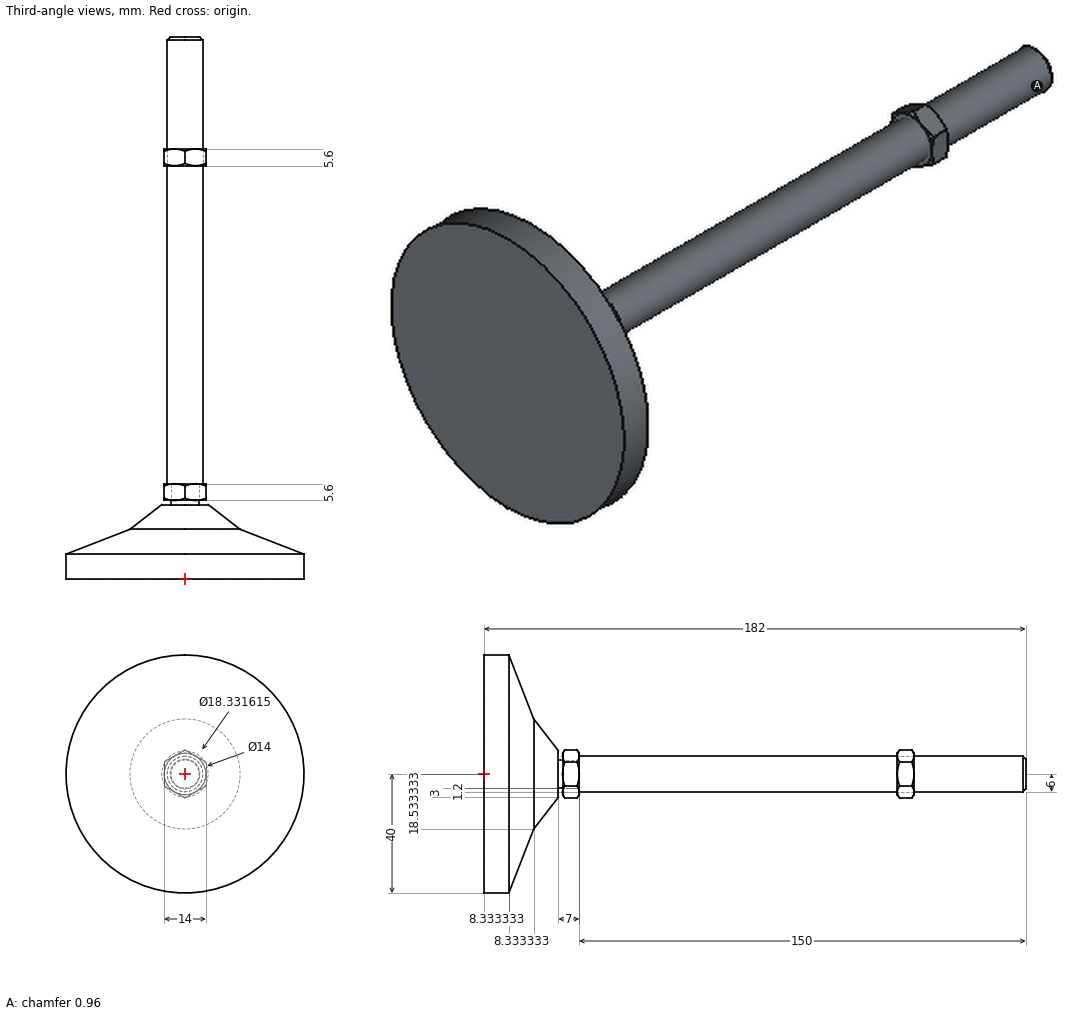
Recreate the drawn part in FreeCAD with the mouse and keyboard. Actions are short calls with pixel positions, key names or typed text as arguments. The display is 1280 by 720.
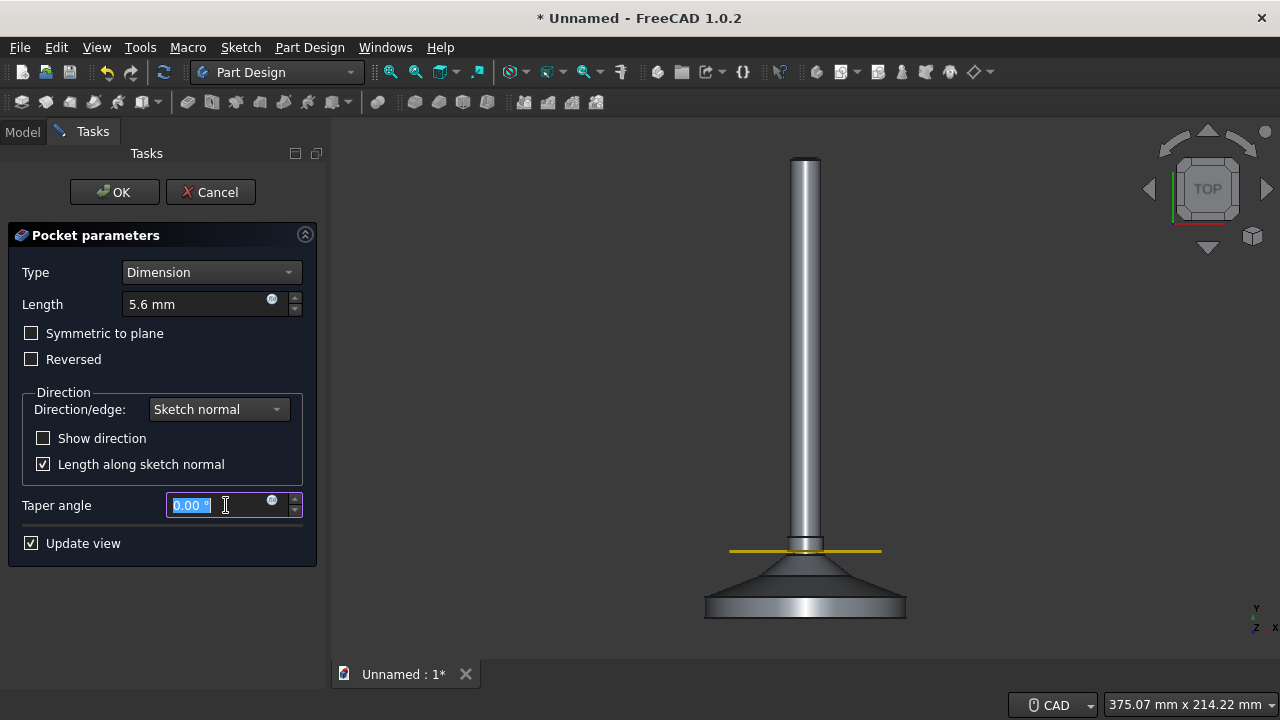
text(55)
key(Tab)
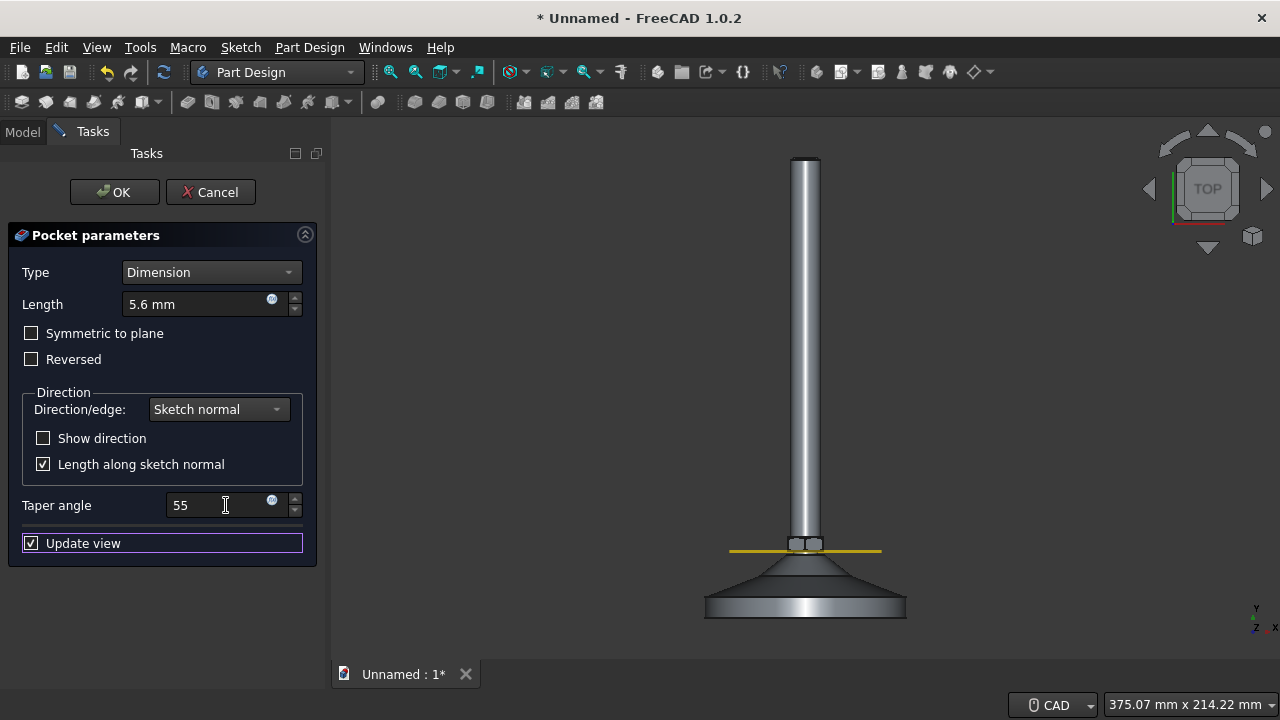
click(115, 192)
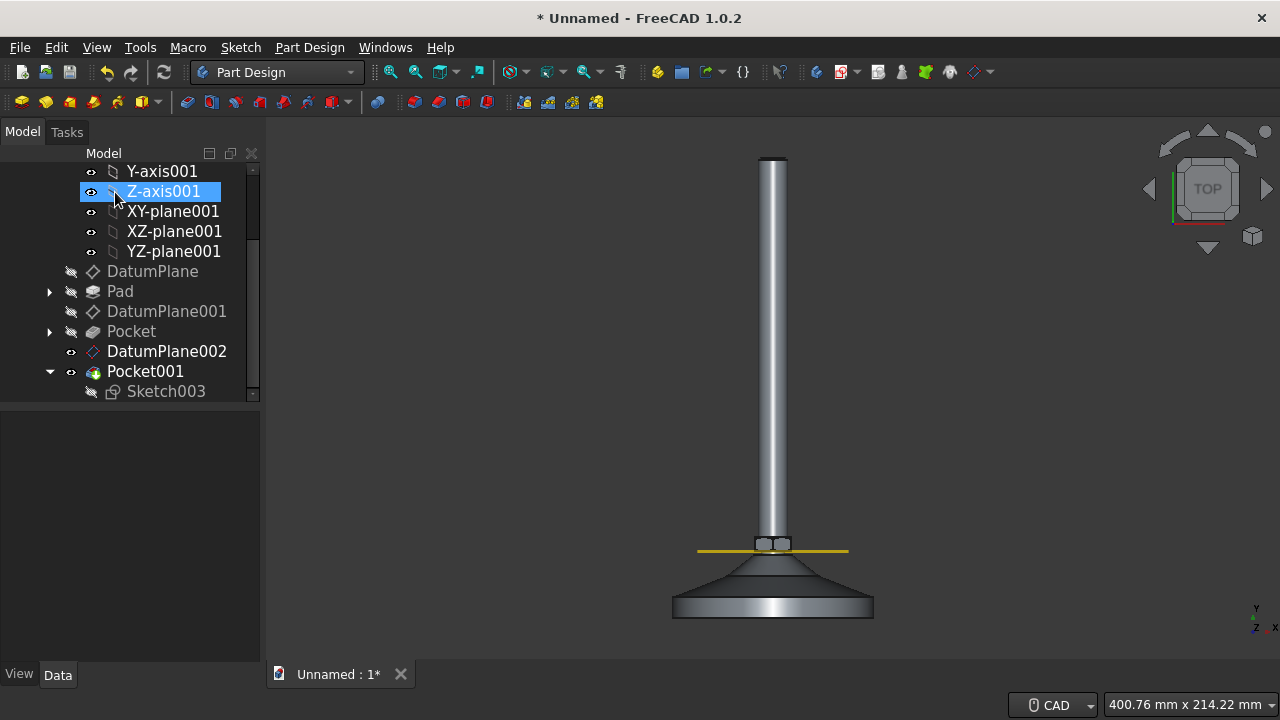
click(116, 352)
key(space)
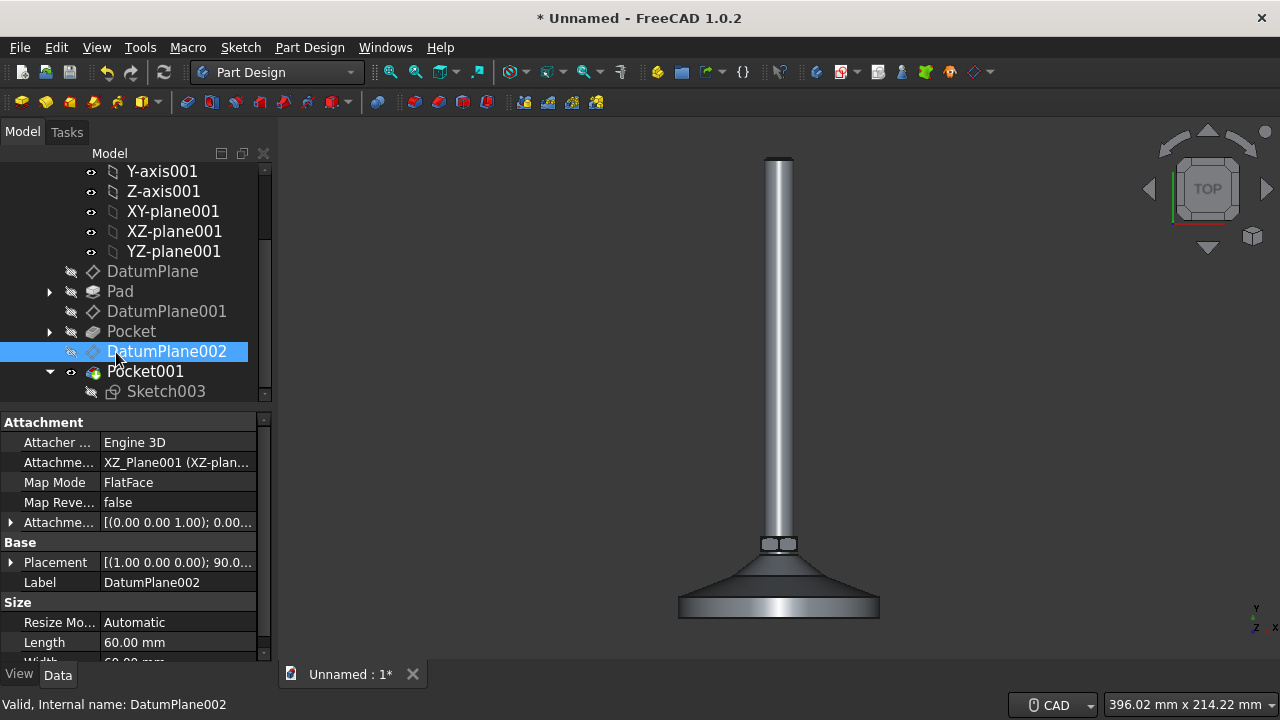
click(392, 72)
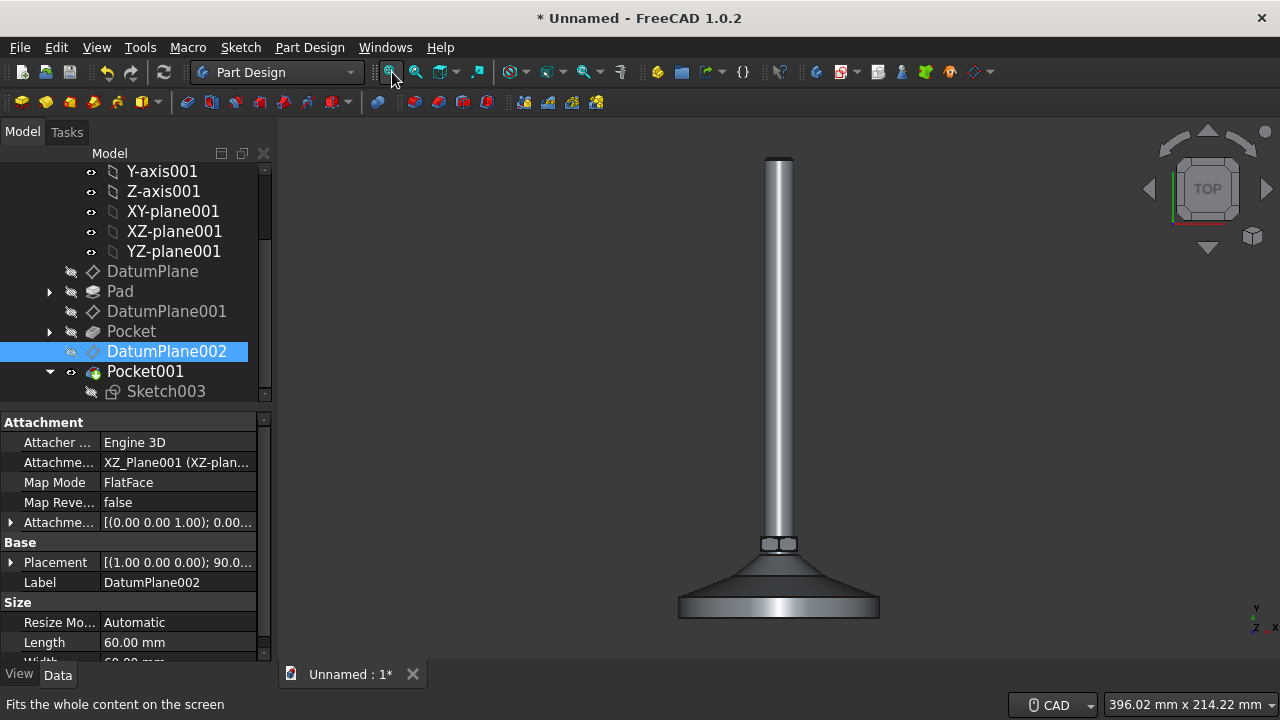
click(318, 619)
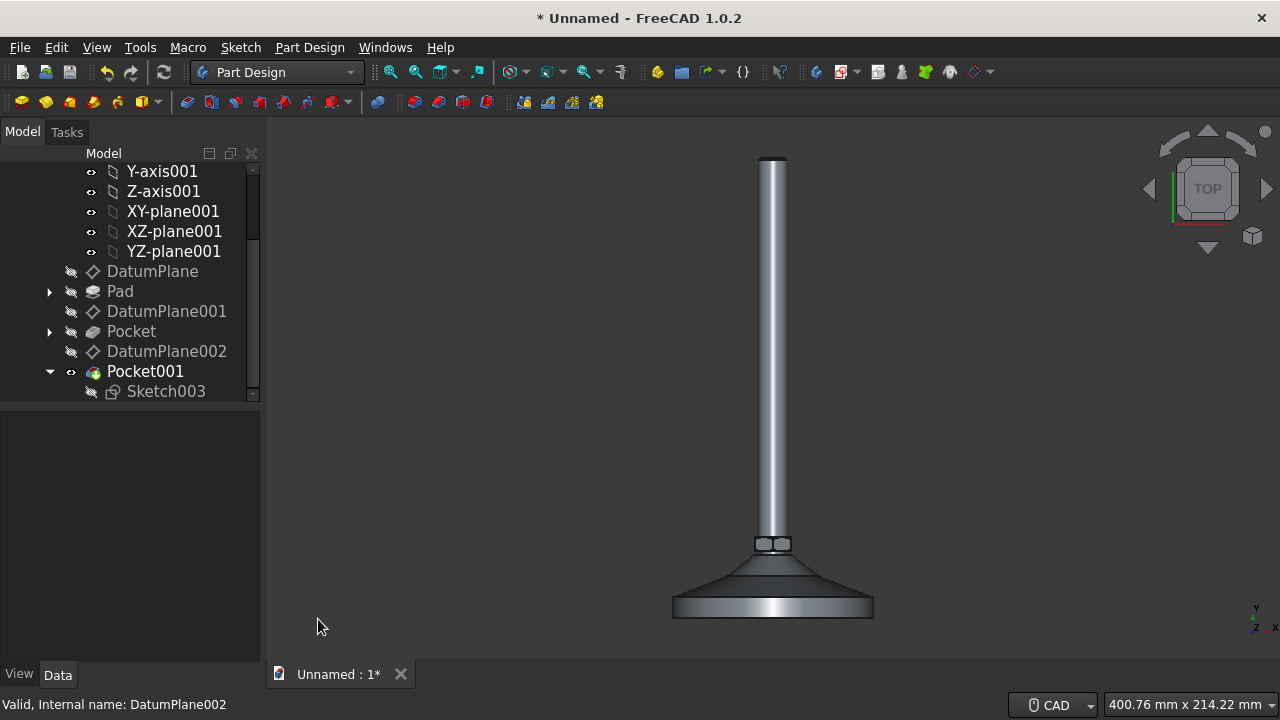
click(818, 72)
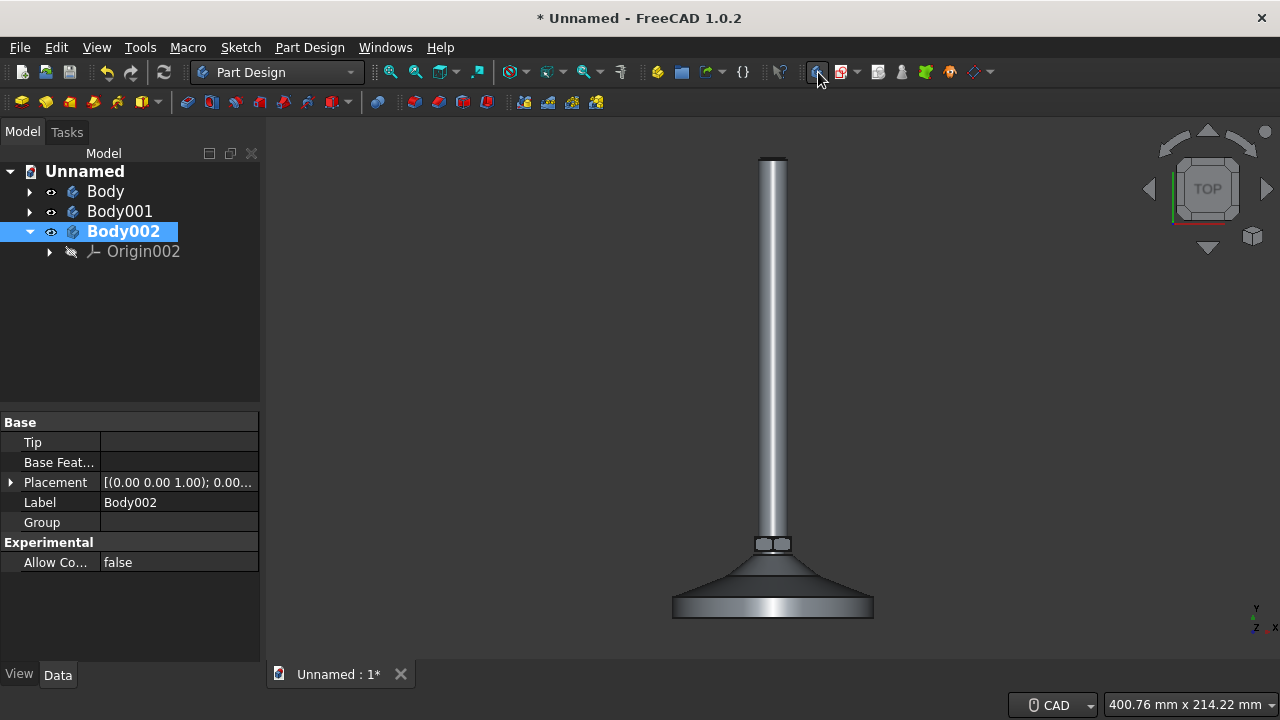
click(50, 252)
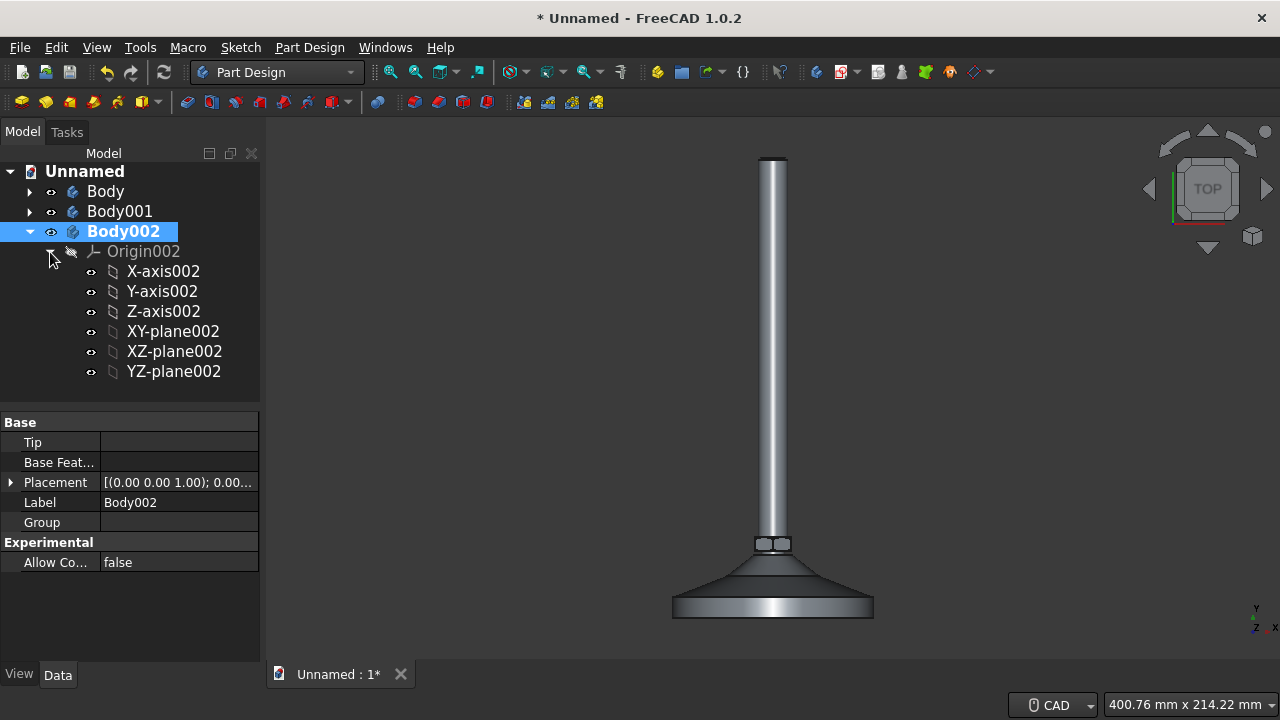
click(136, 352)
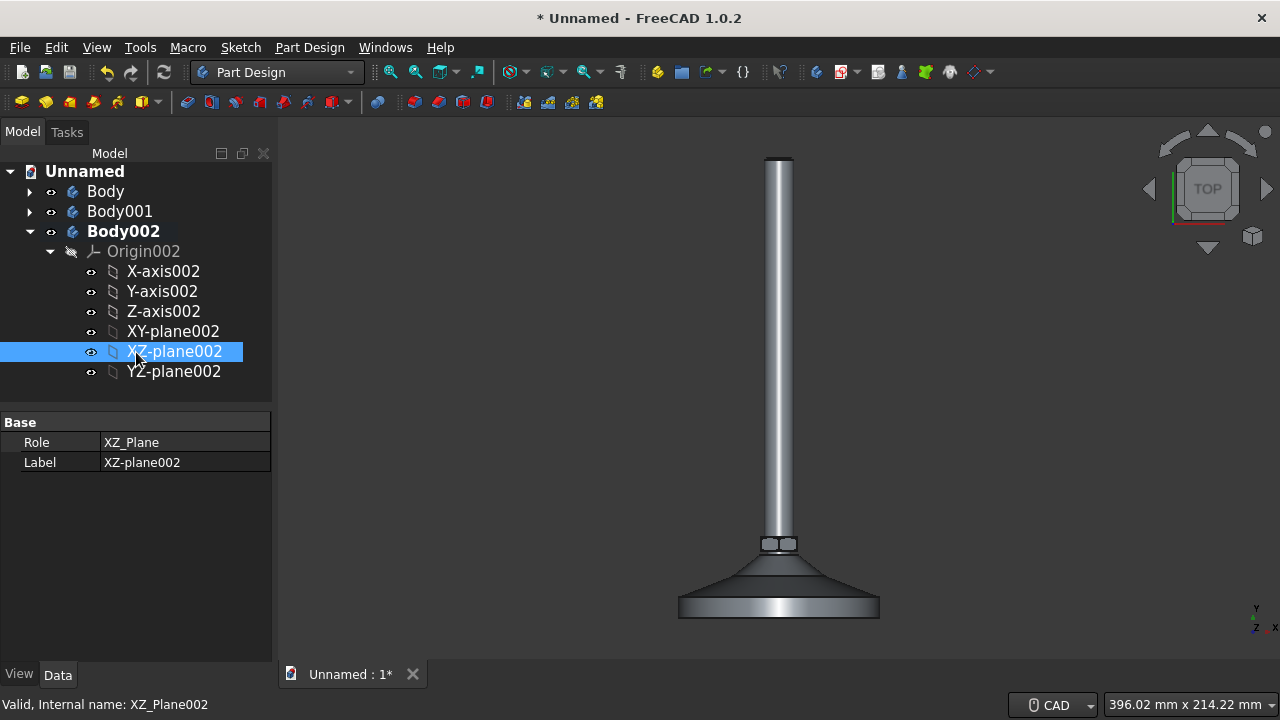
click(974, 72)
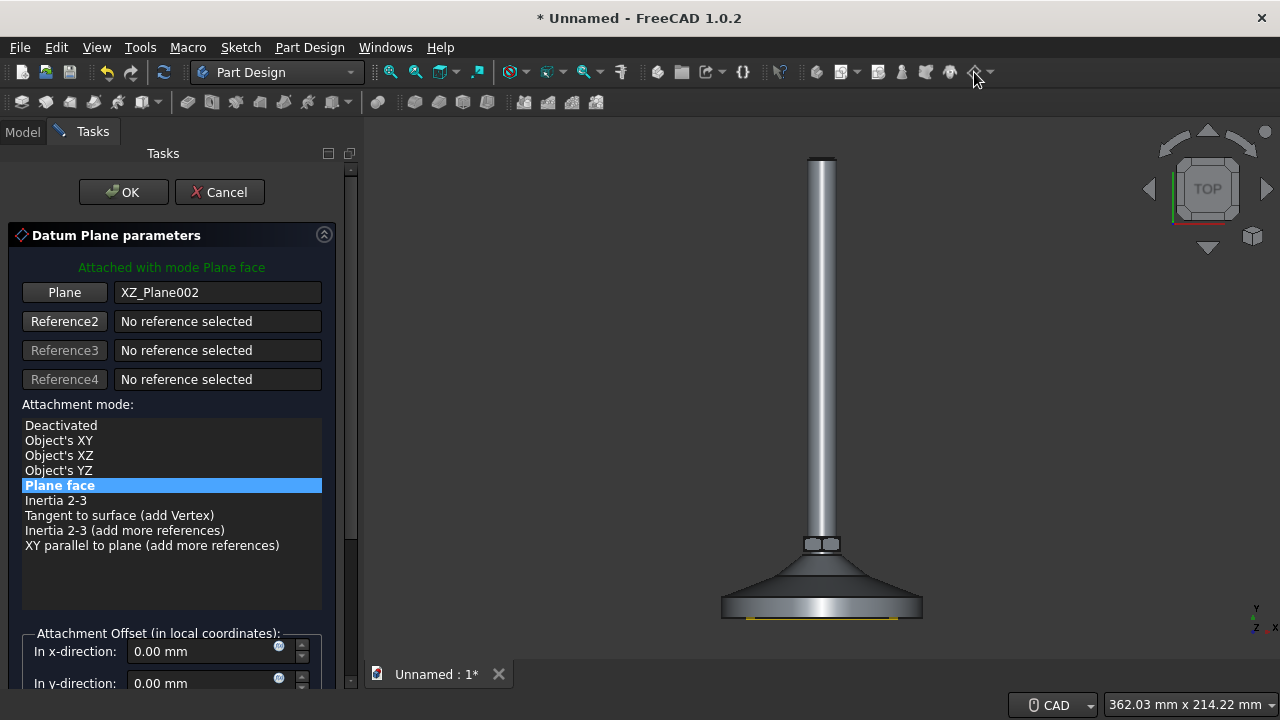
scroll(351, 426, down, 2)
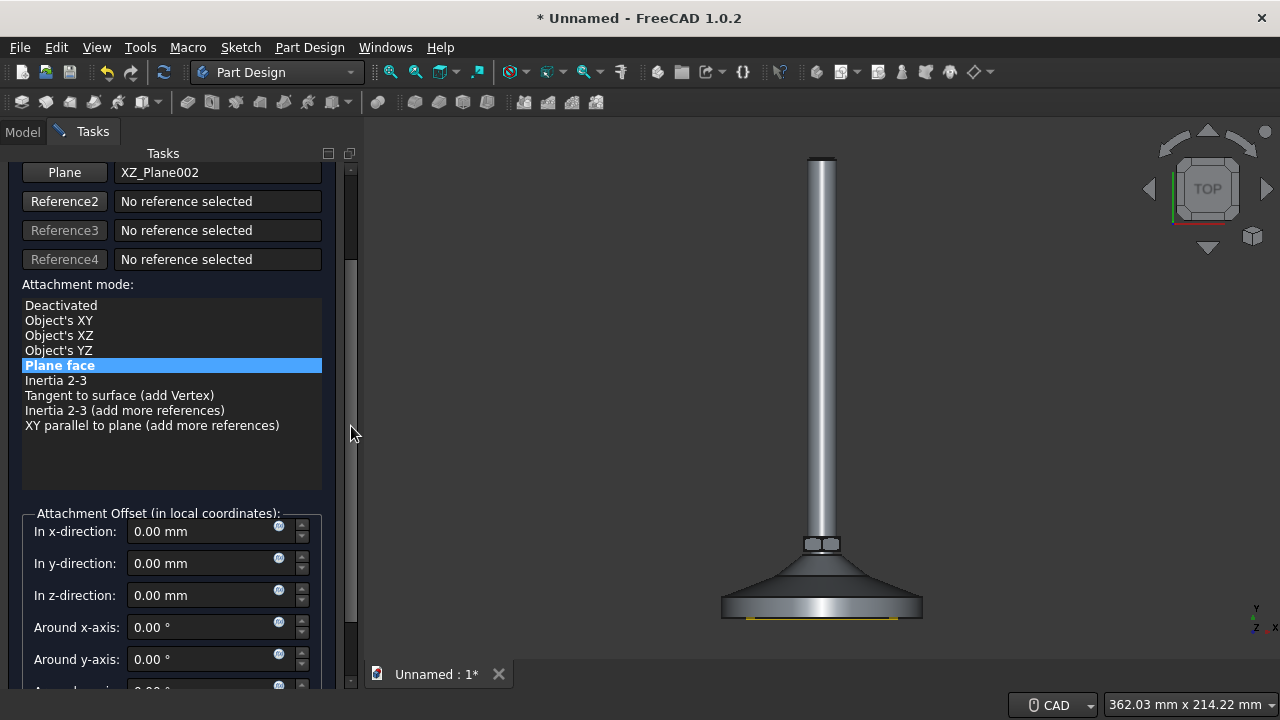
triple_click(210, 595)